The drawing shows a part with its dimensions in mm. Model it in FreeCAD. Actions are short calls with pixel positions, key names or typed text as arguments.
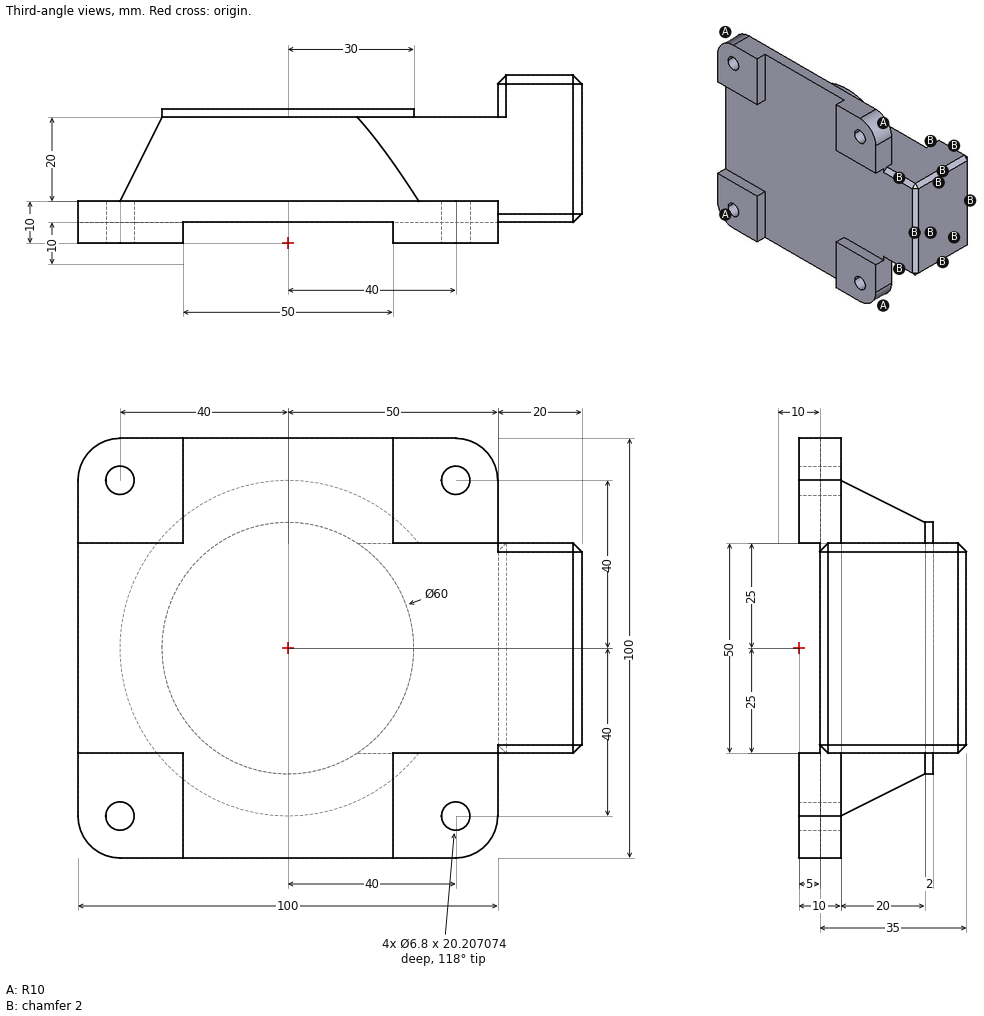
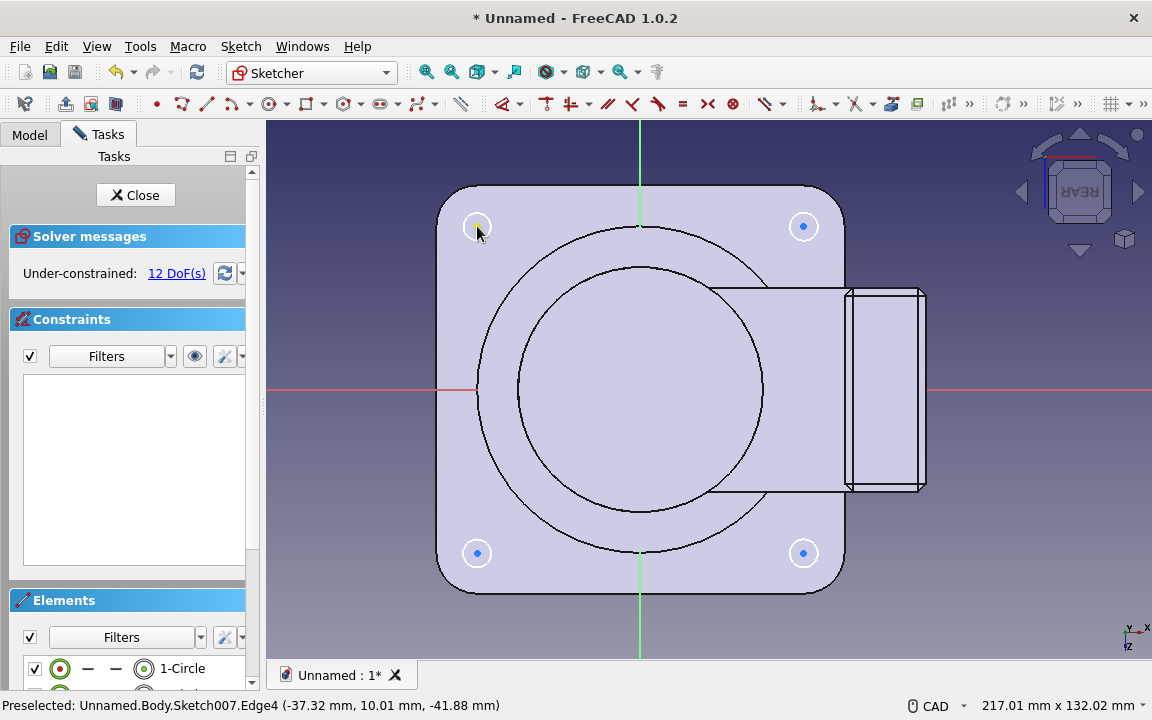
click(814, 217)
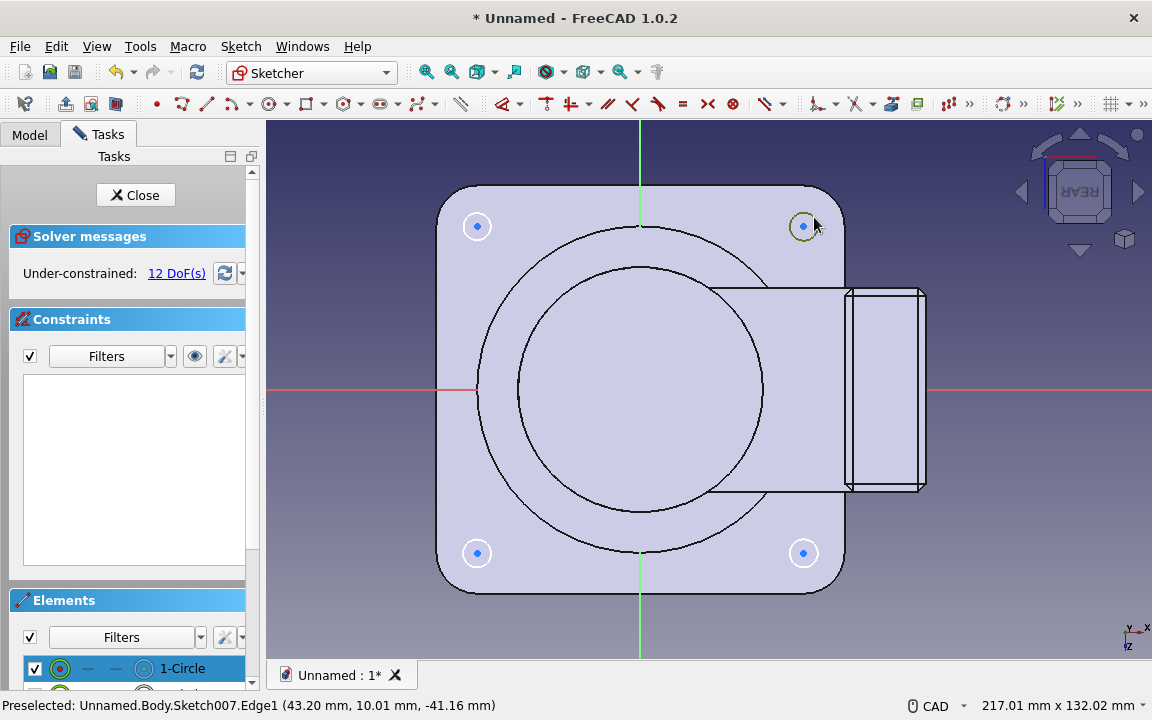
click(814, 543)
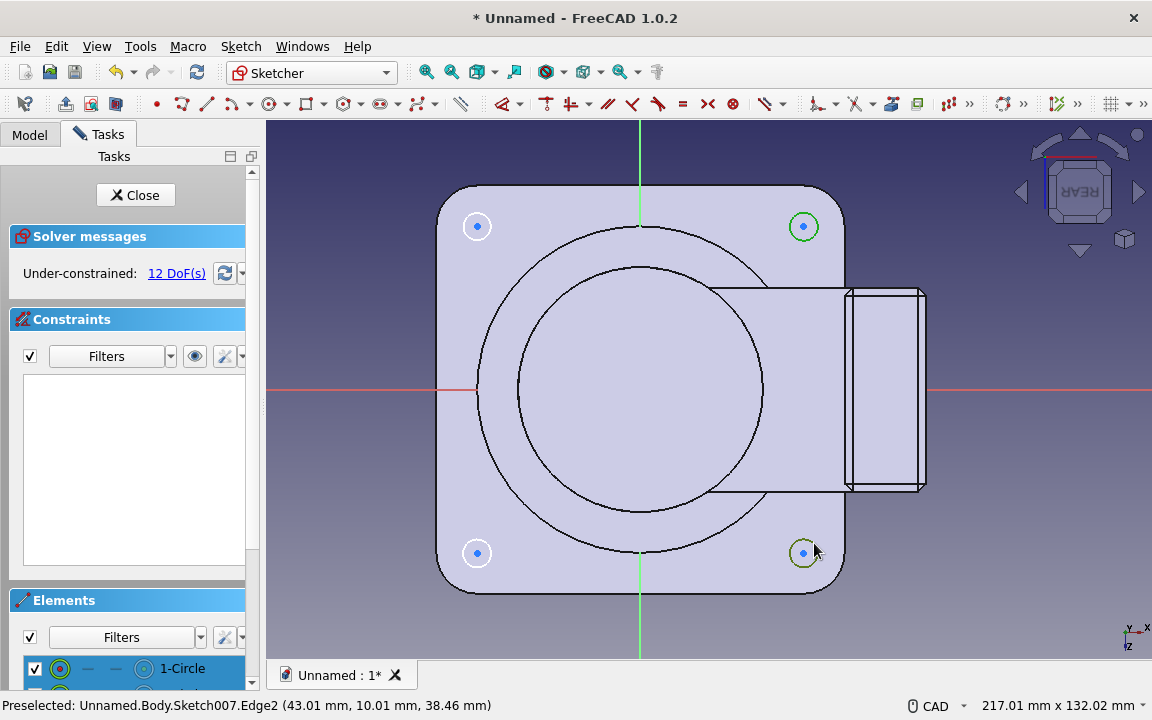
click(487, 544)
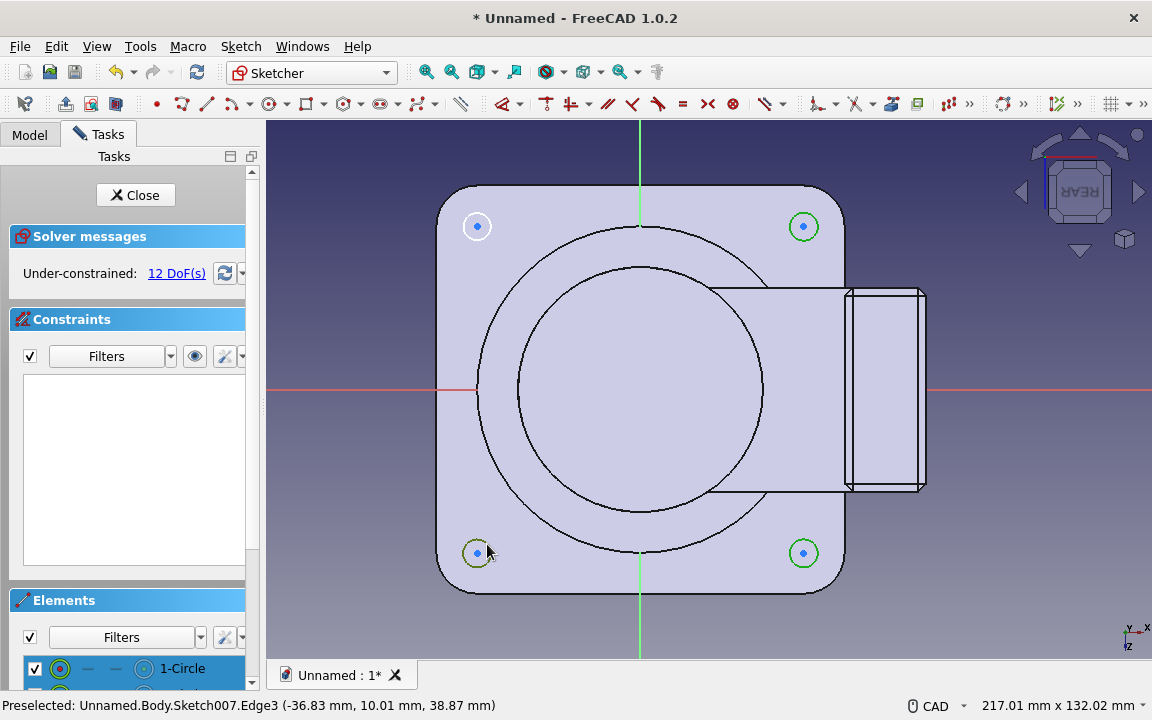
click(487, 217)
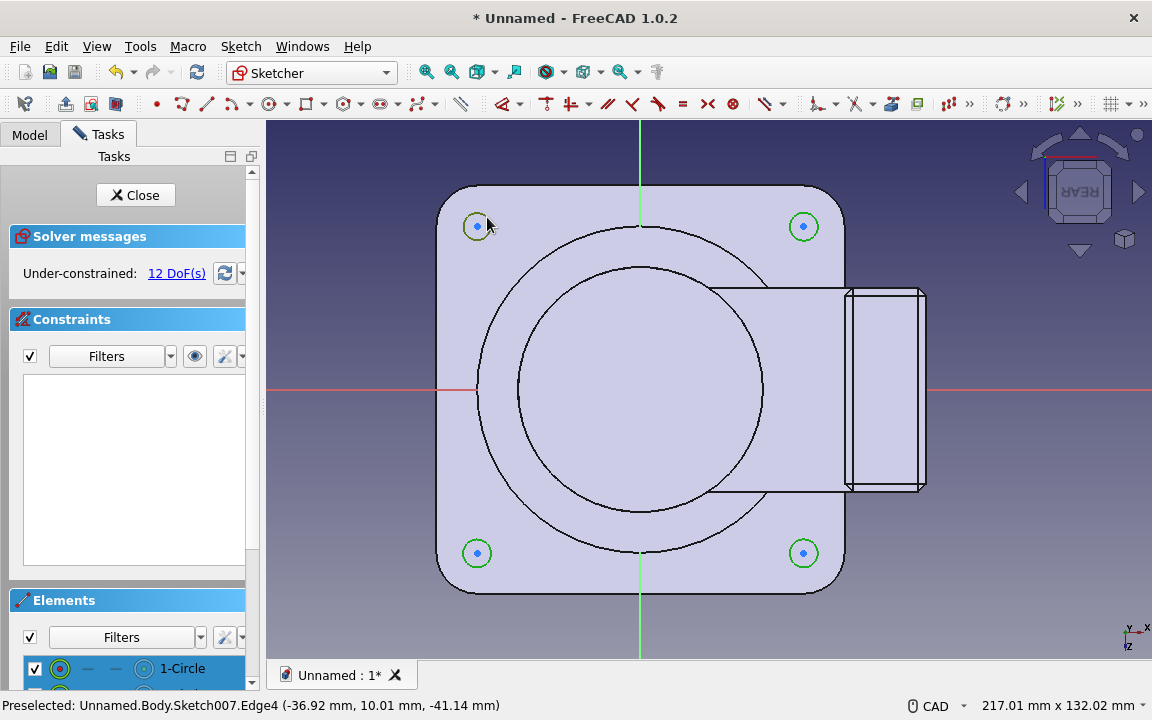
key(e)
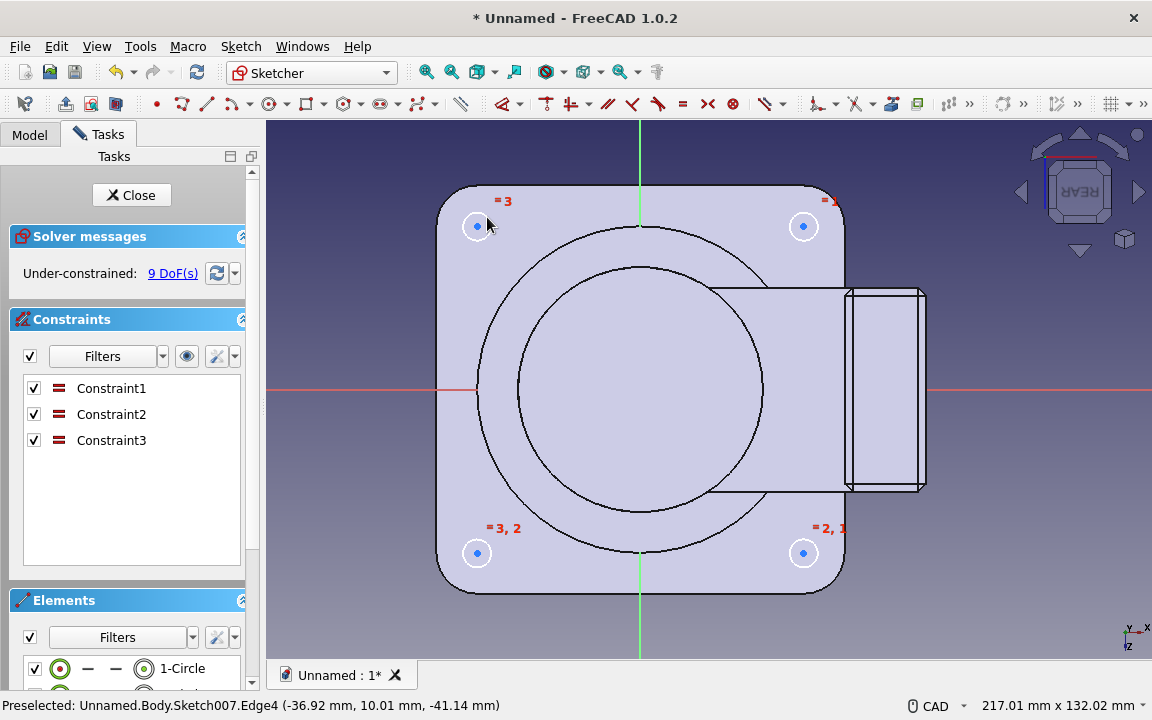
click(804, 227)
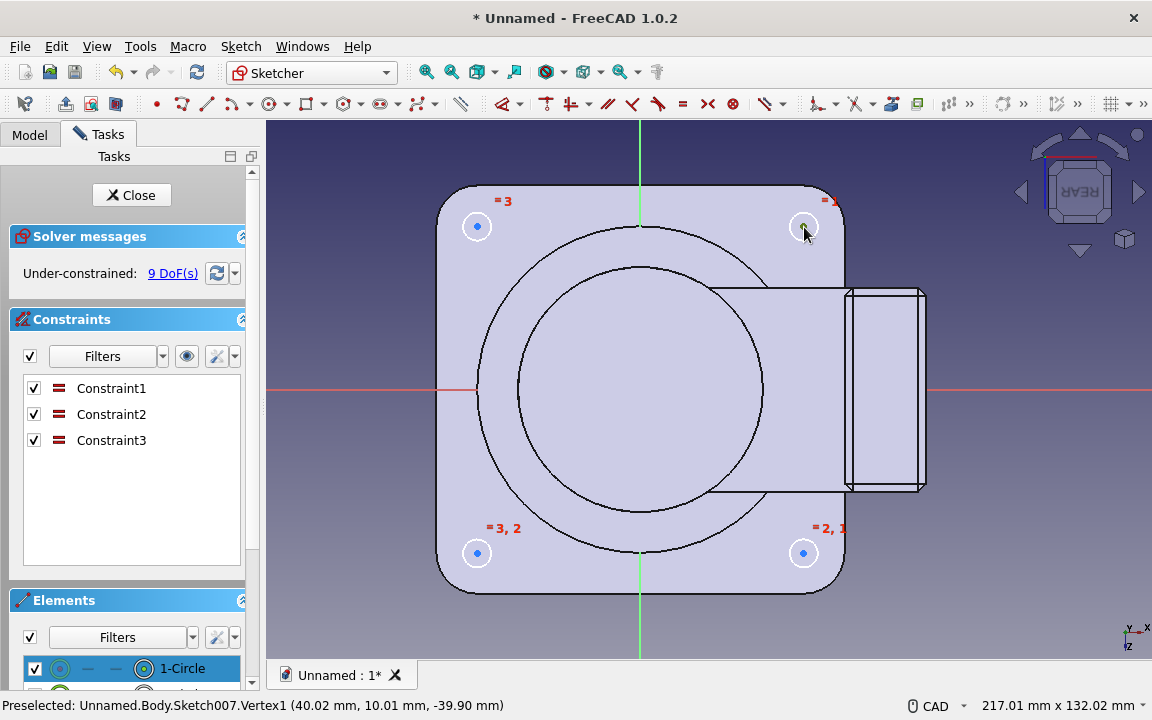
click(804, 553)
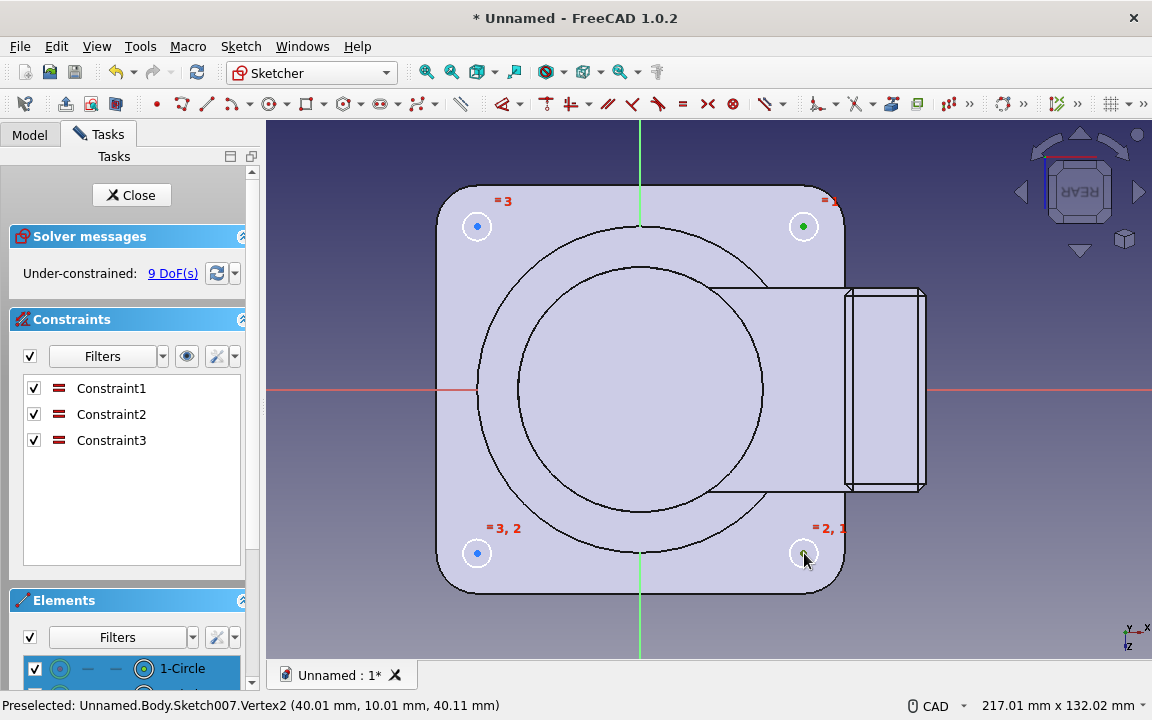
key(v)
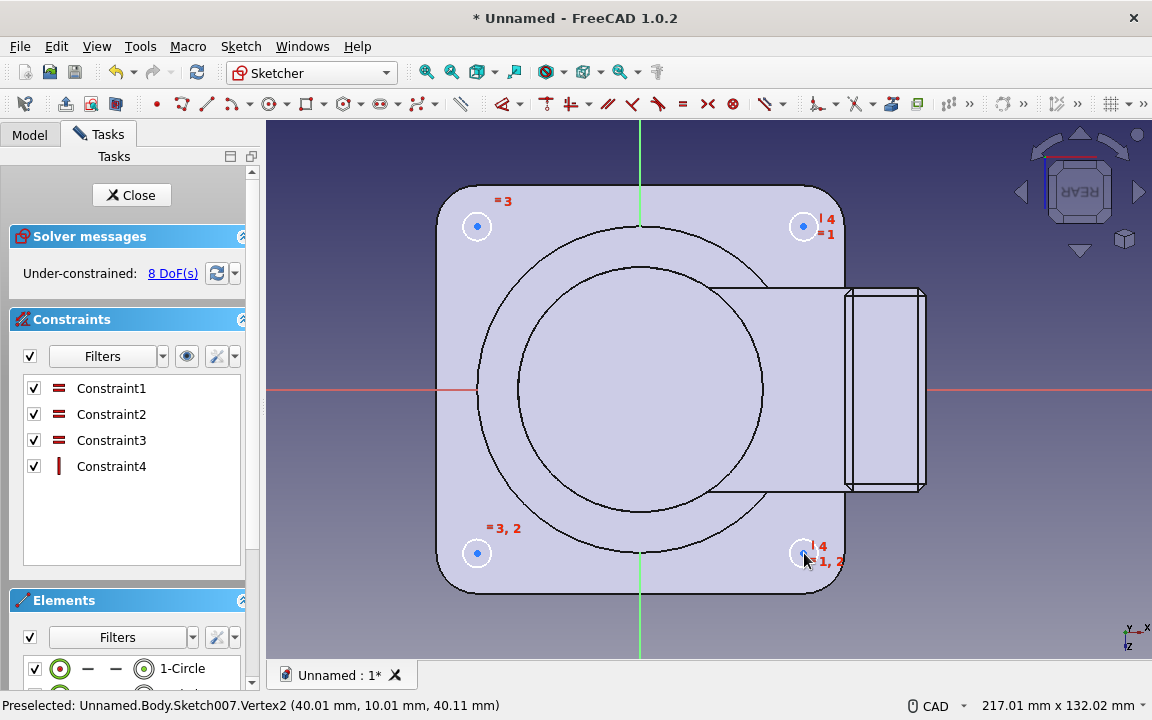
click(804, 553)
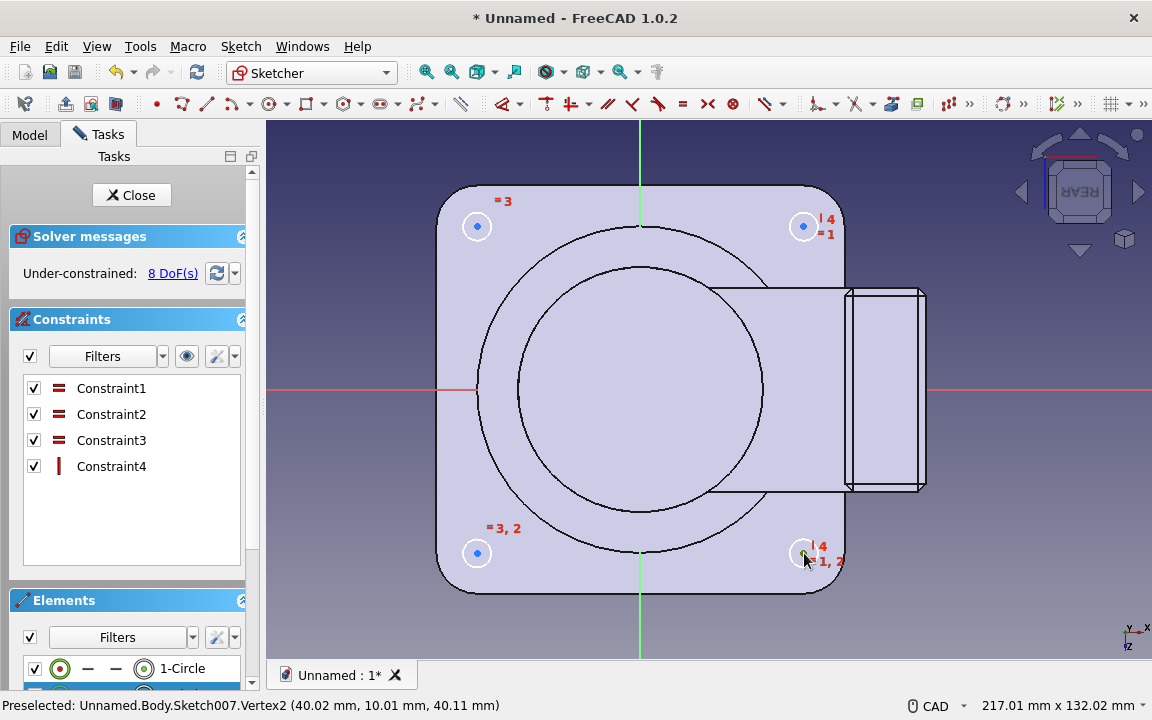
click(477, 553)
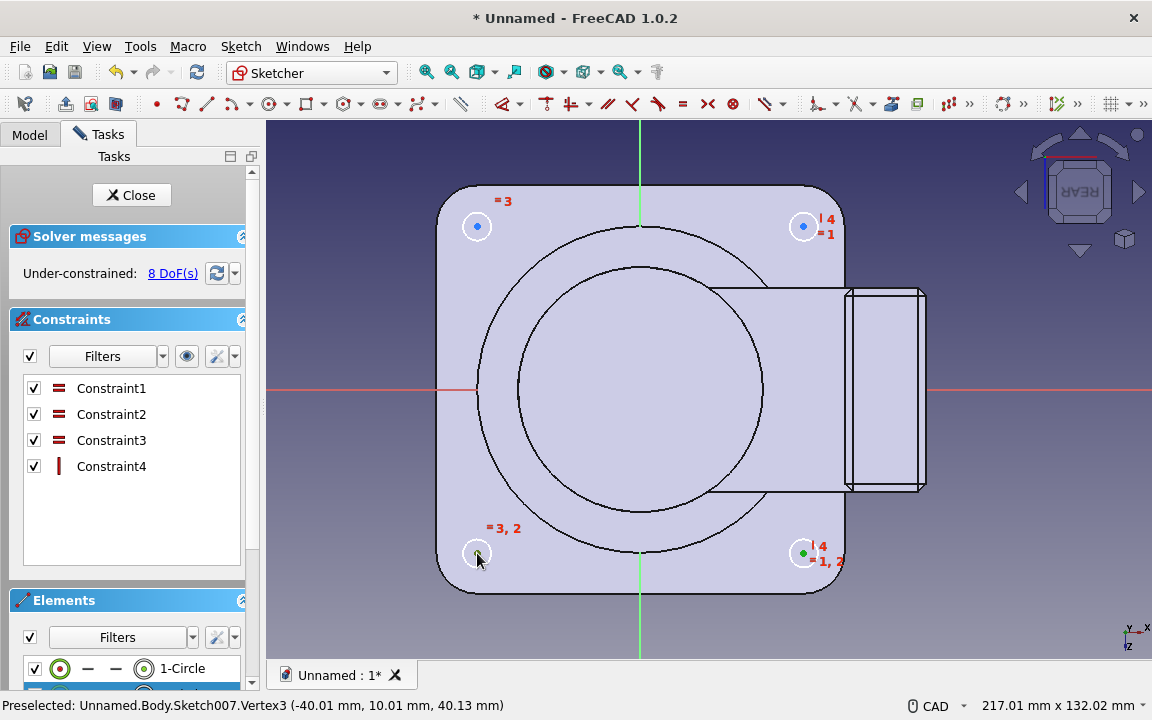
click(588, 104)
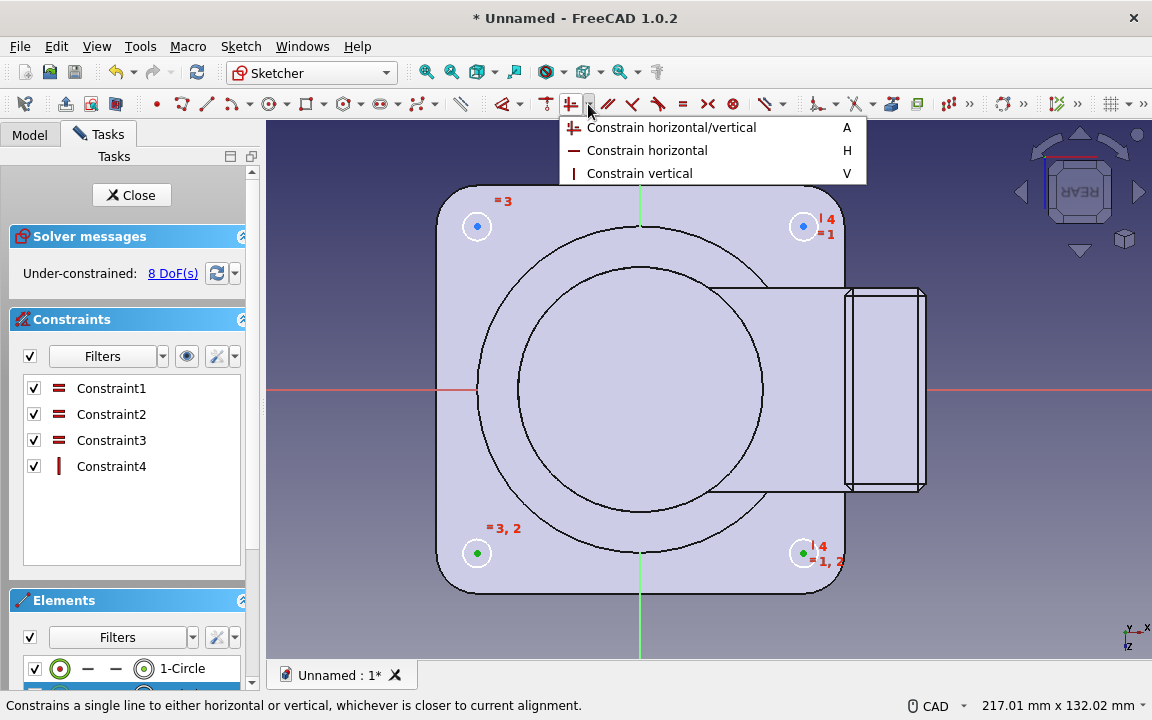
click(713, 150)